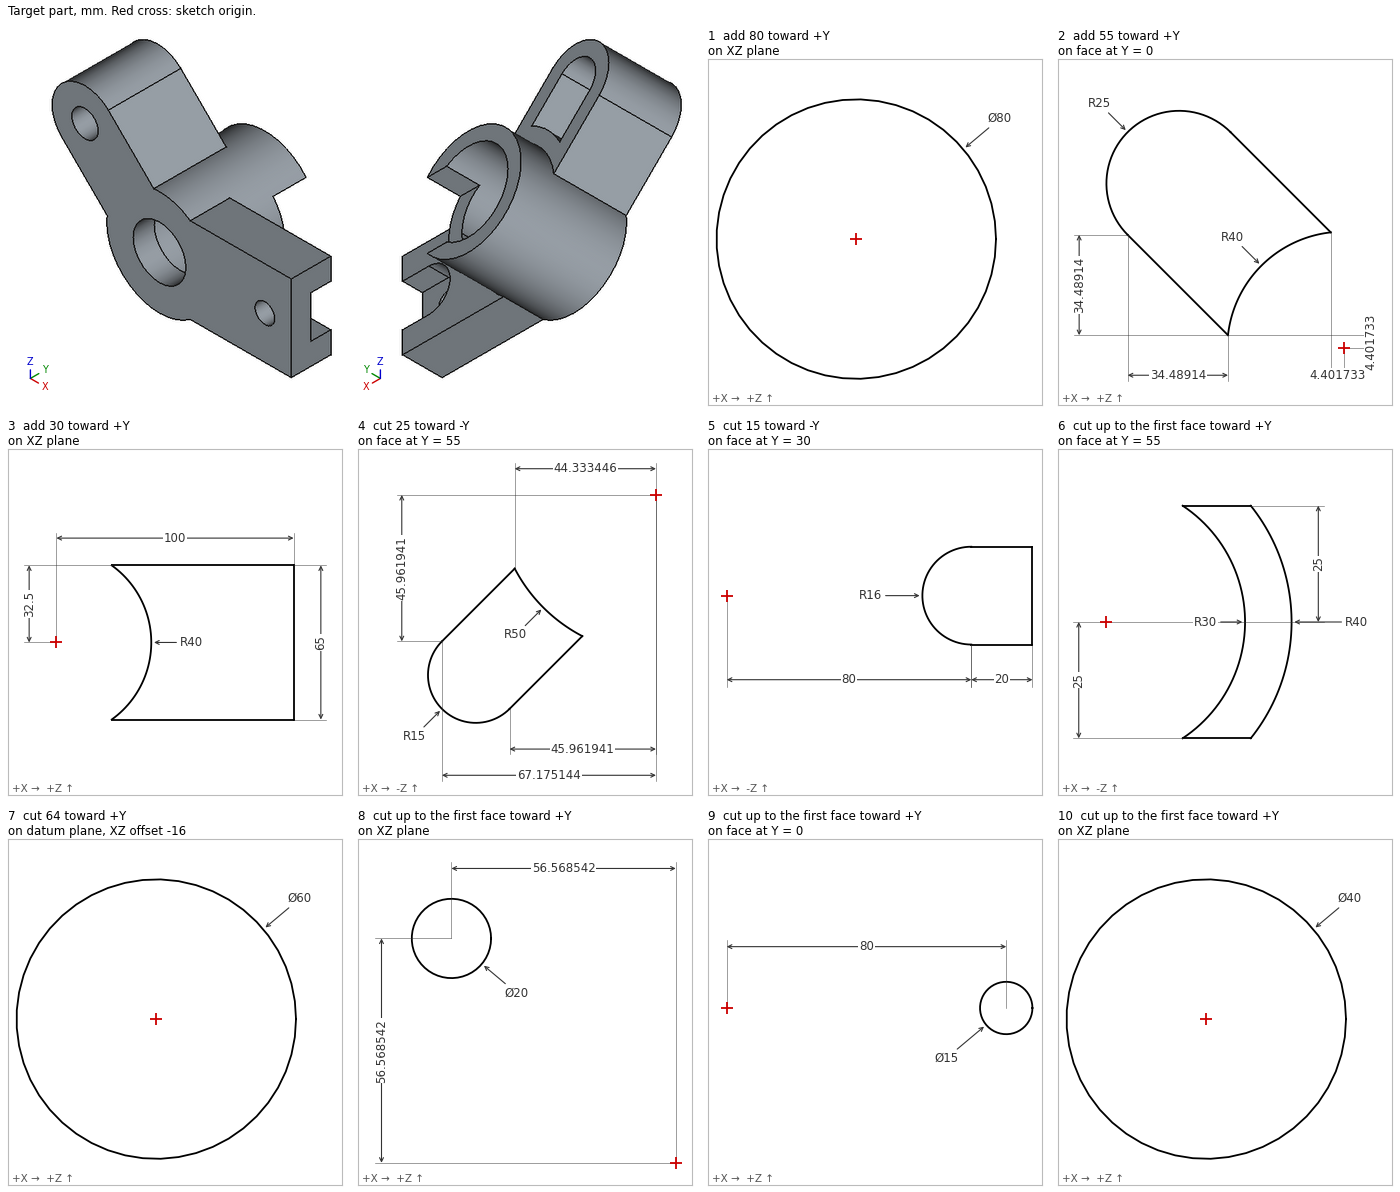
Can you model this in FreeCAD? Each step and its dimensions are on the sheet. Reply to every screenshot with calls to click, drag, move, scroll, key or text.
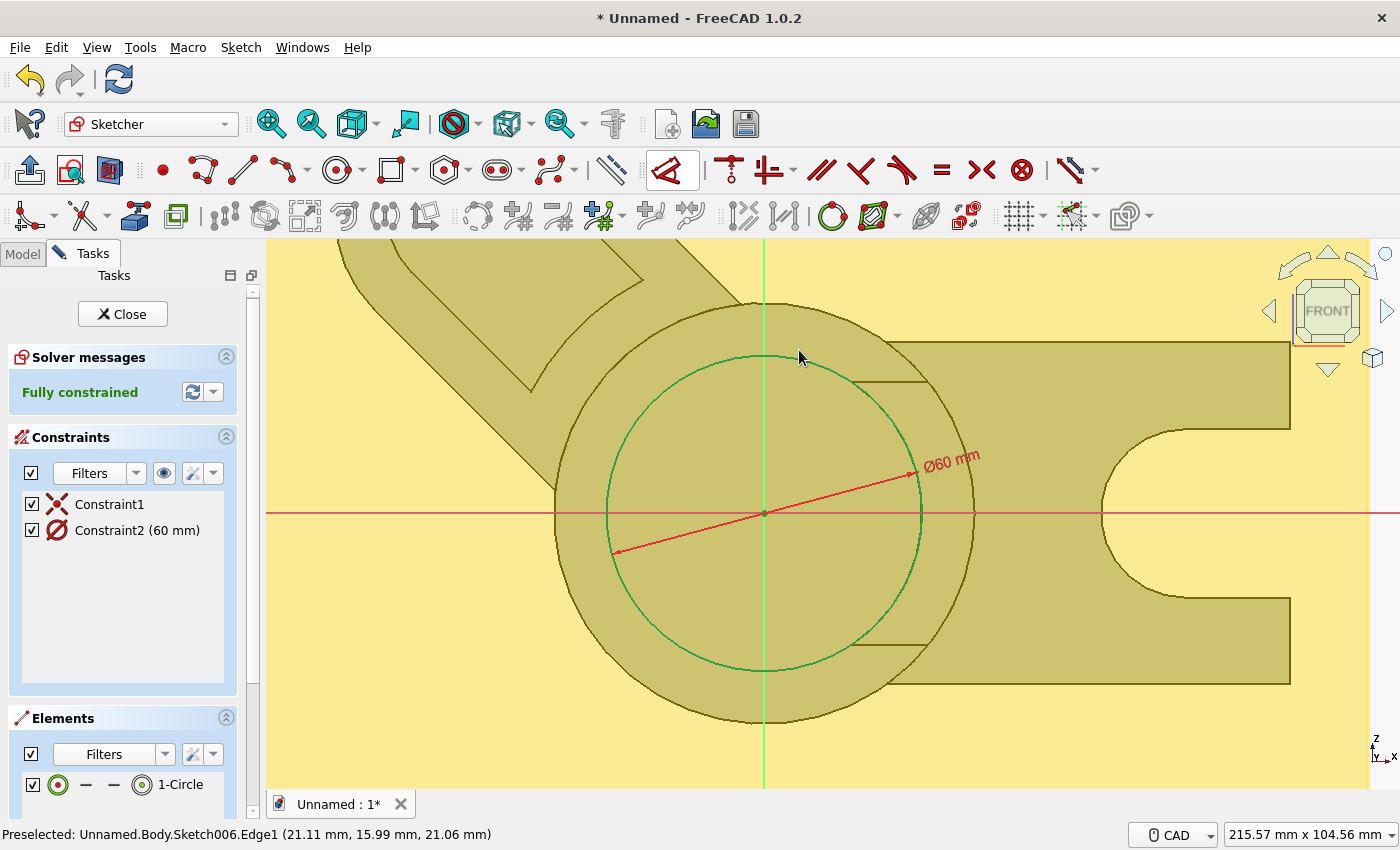
click(123, 314)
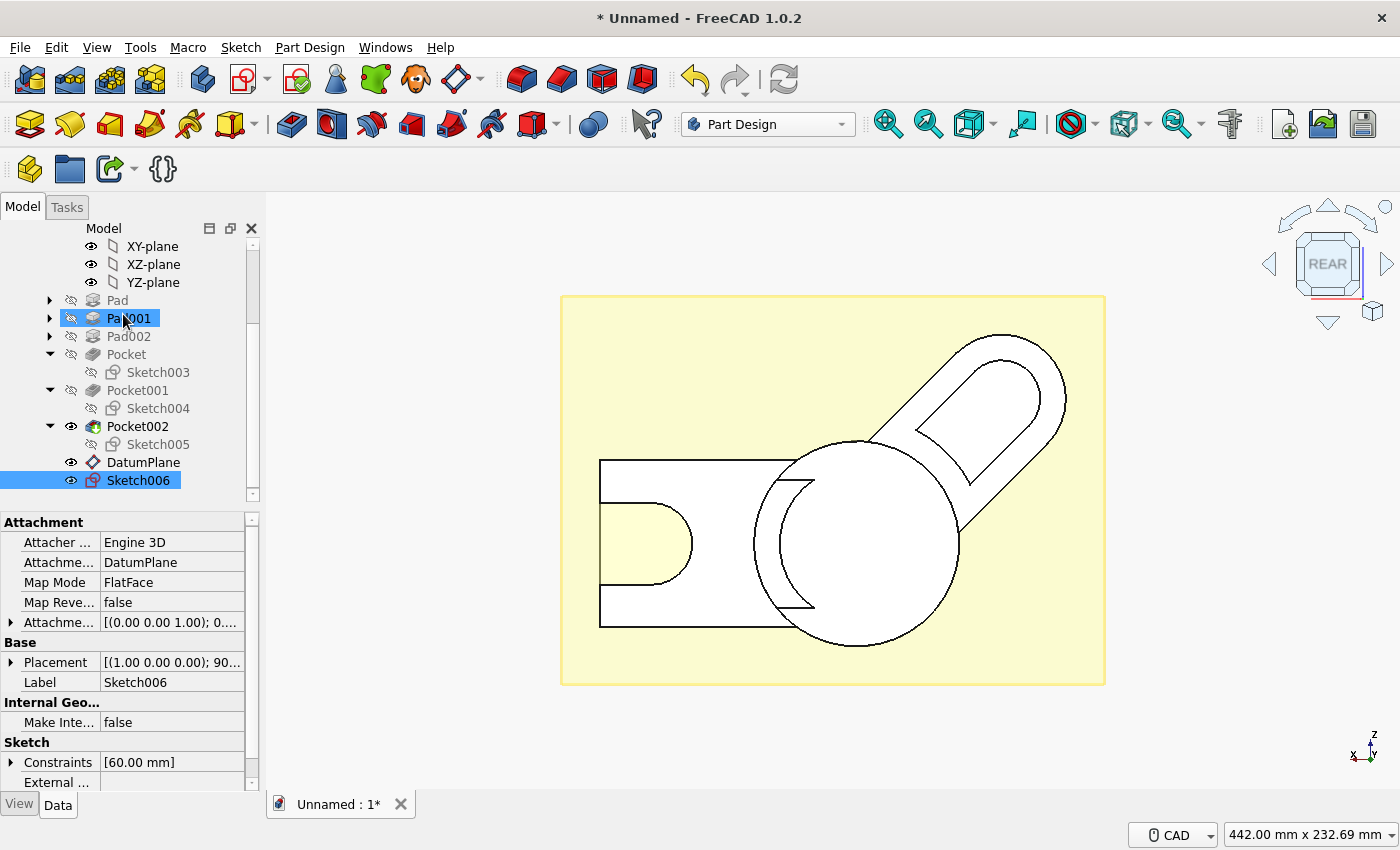
click(292, 124)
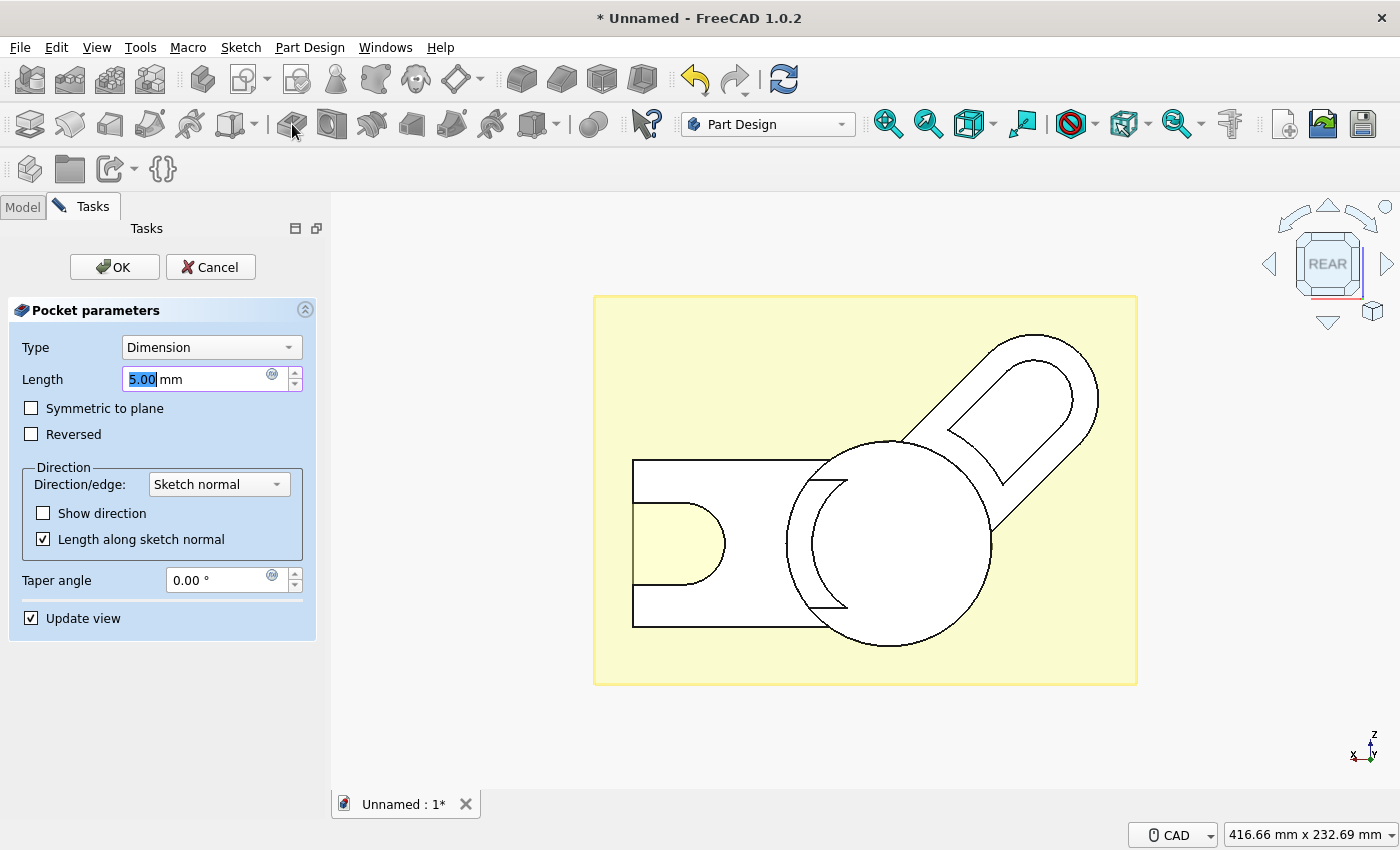
text(64)
key(Tab)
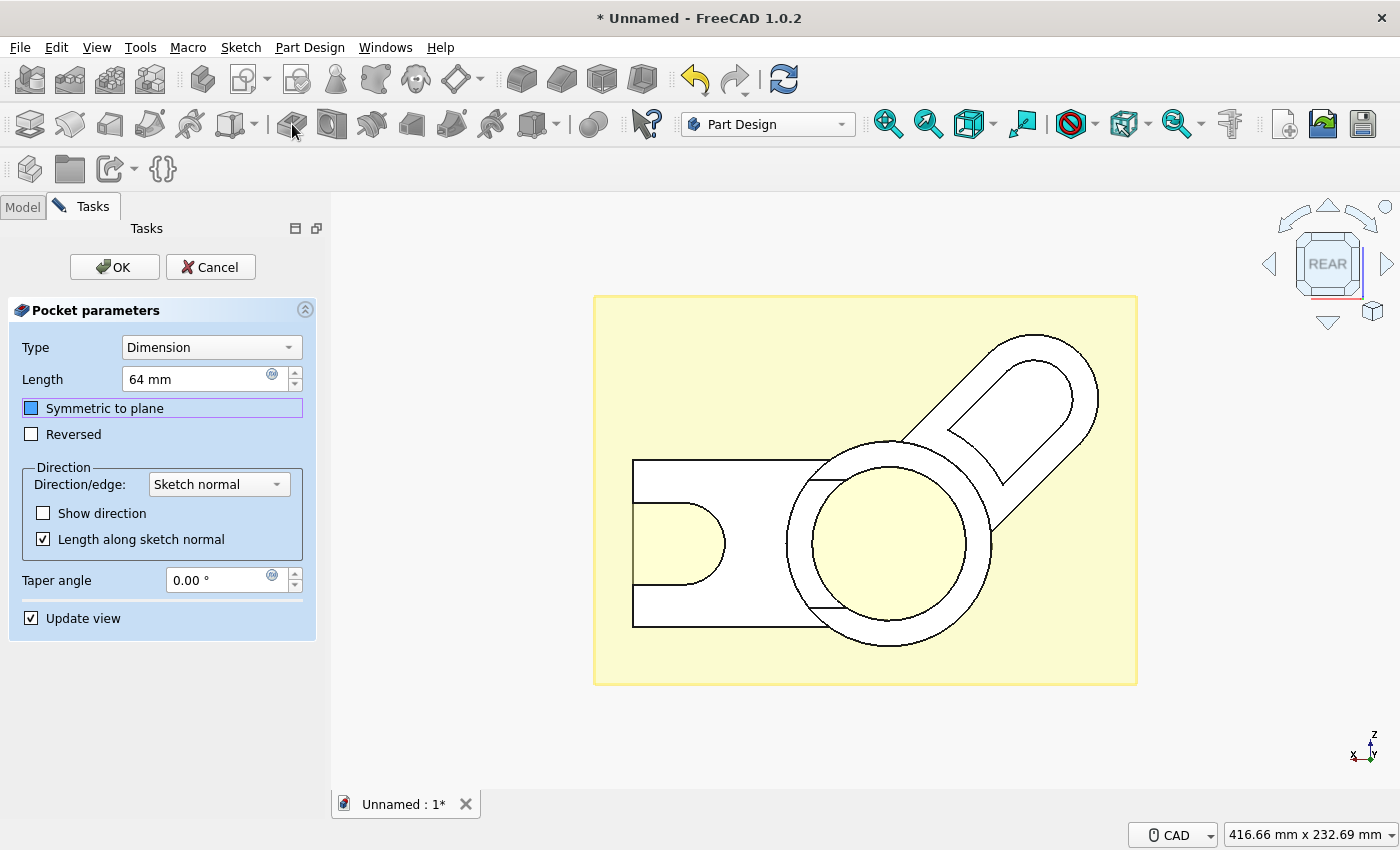
click(115, 267)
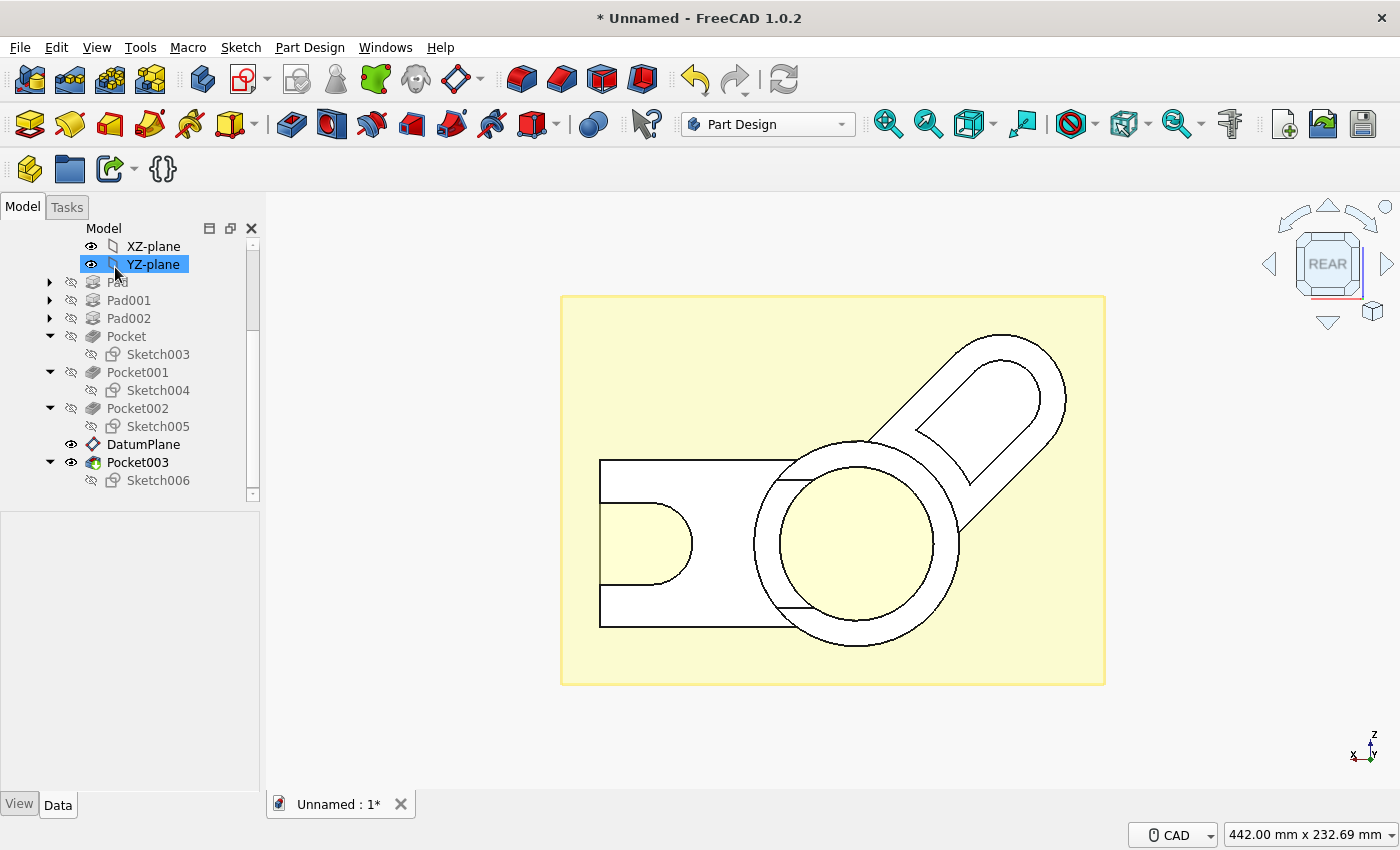
click(116, 444)
key(space)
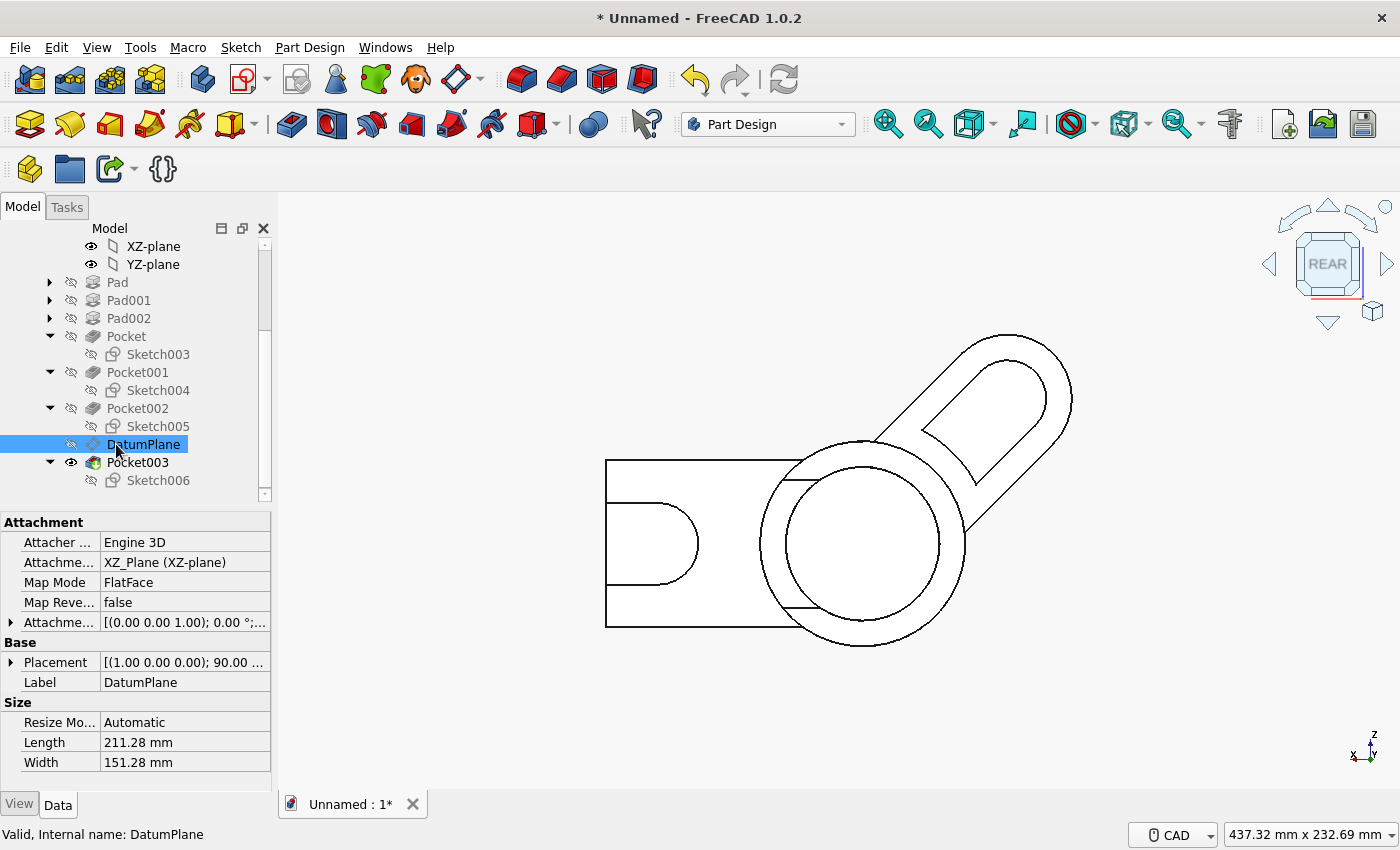
click(318, 749)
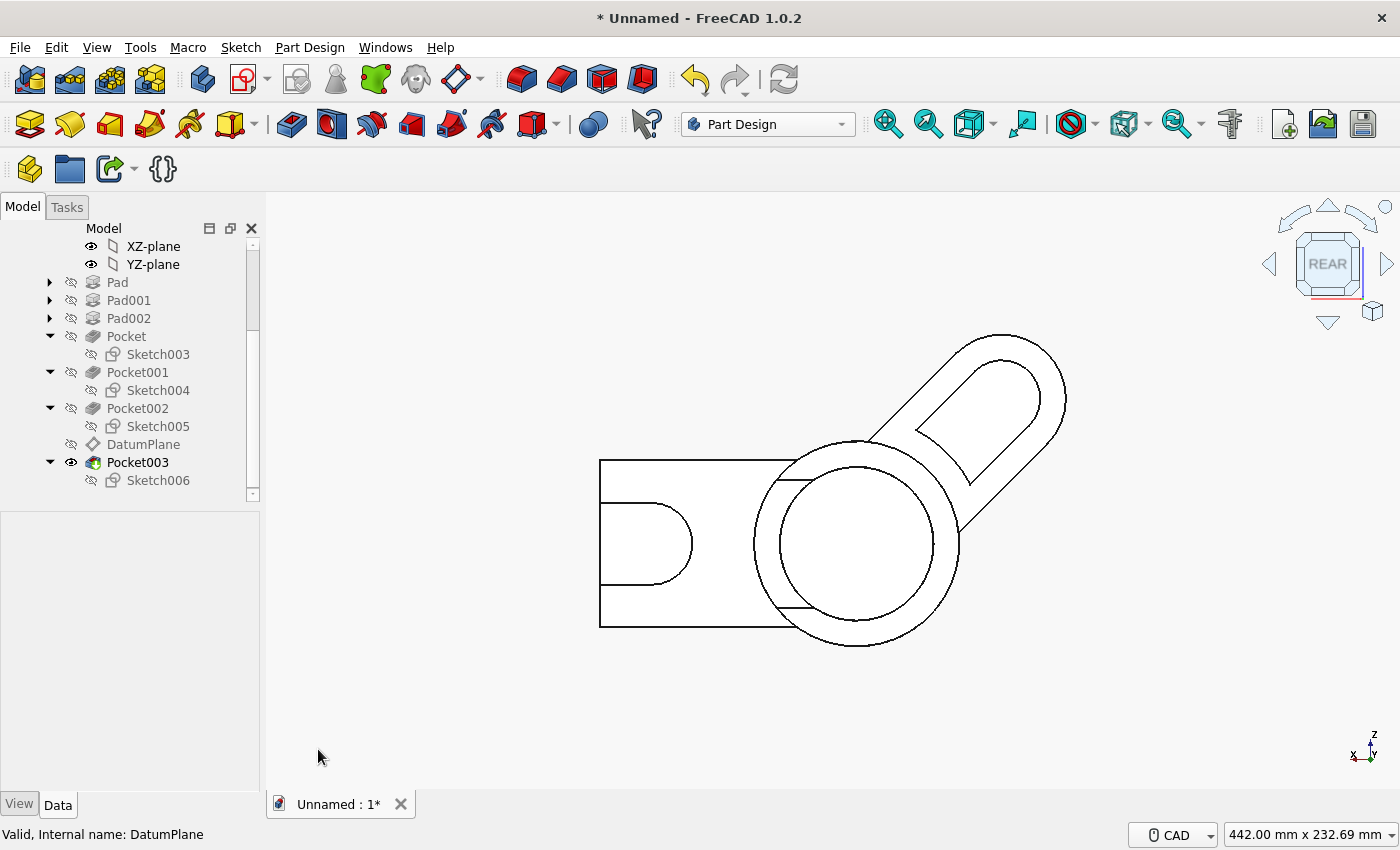
click(244, 80)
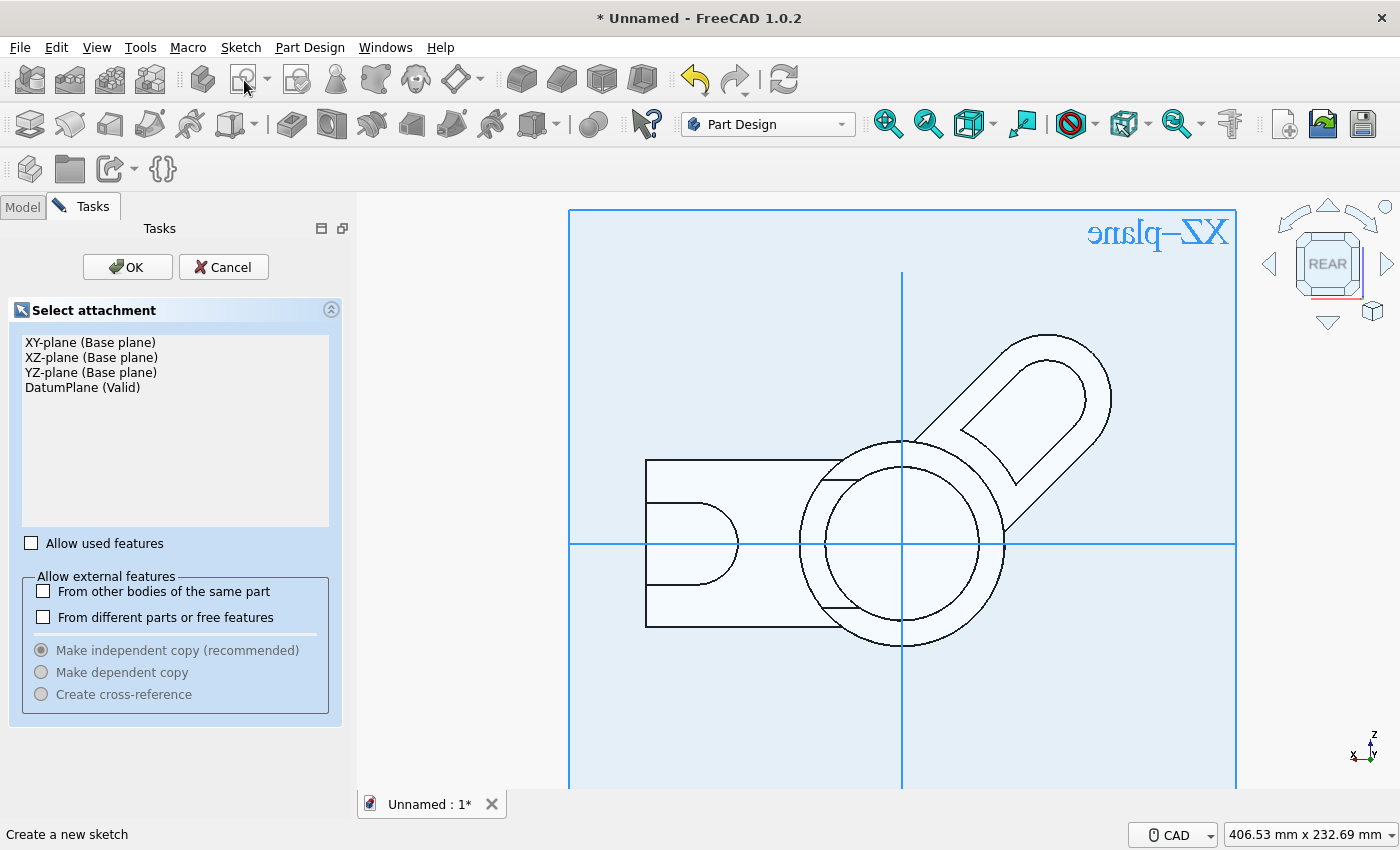
click(82, 358)